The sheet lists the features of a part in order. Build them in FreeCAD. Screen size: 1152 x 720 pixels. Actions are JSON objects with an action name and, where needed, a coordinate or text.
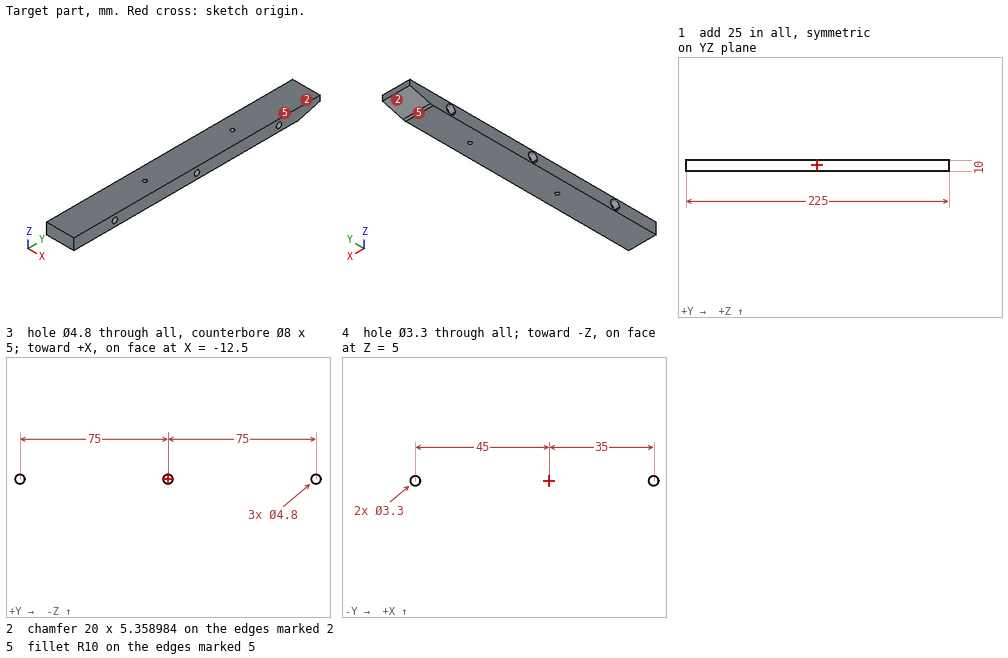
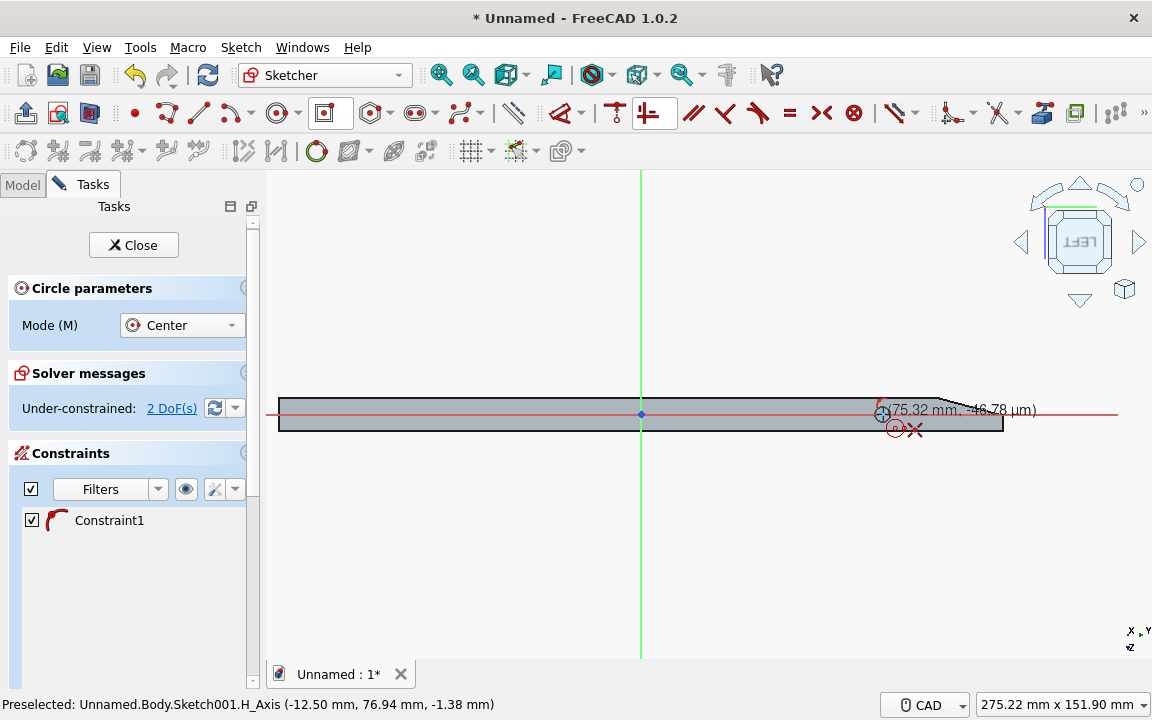
{"action": "scroll", "coordinate": [641, 414], "scroll_direction": "up", "scroll_amount": 6}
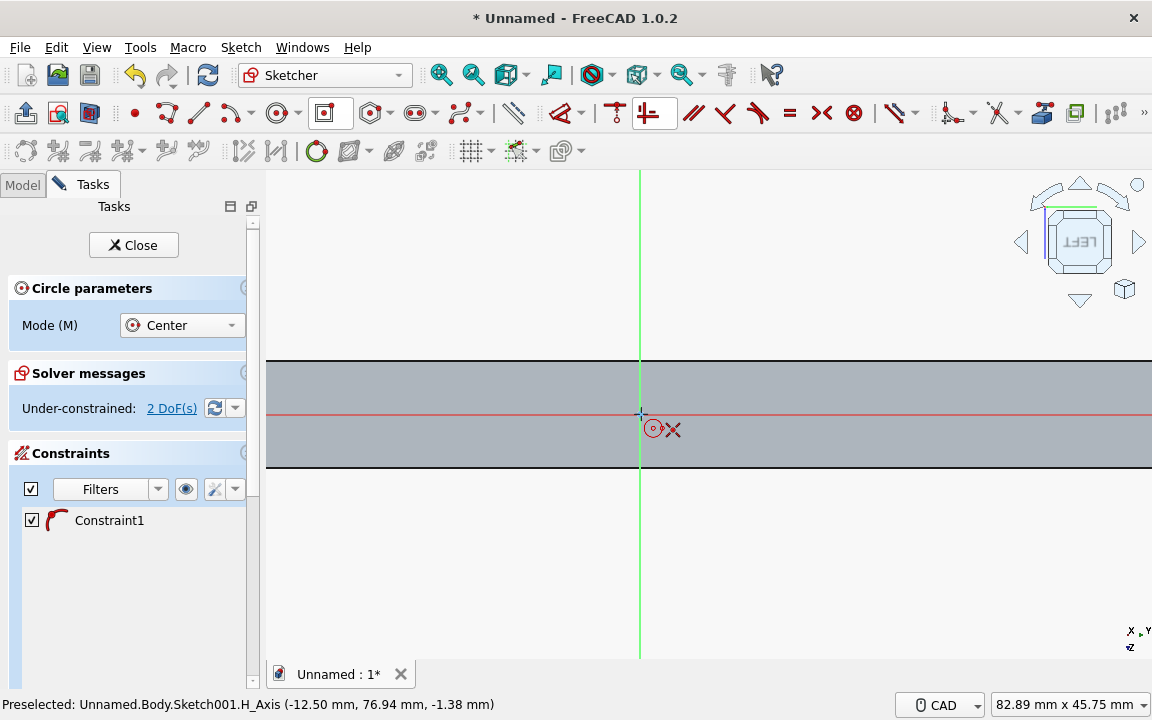
{"action": "left_click", "coordinate": [640, 414]}
{"action": "left_click", "coordinate": [658, 396]}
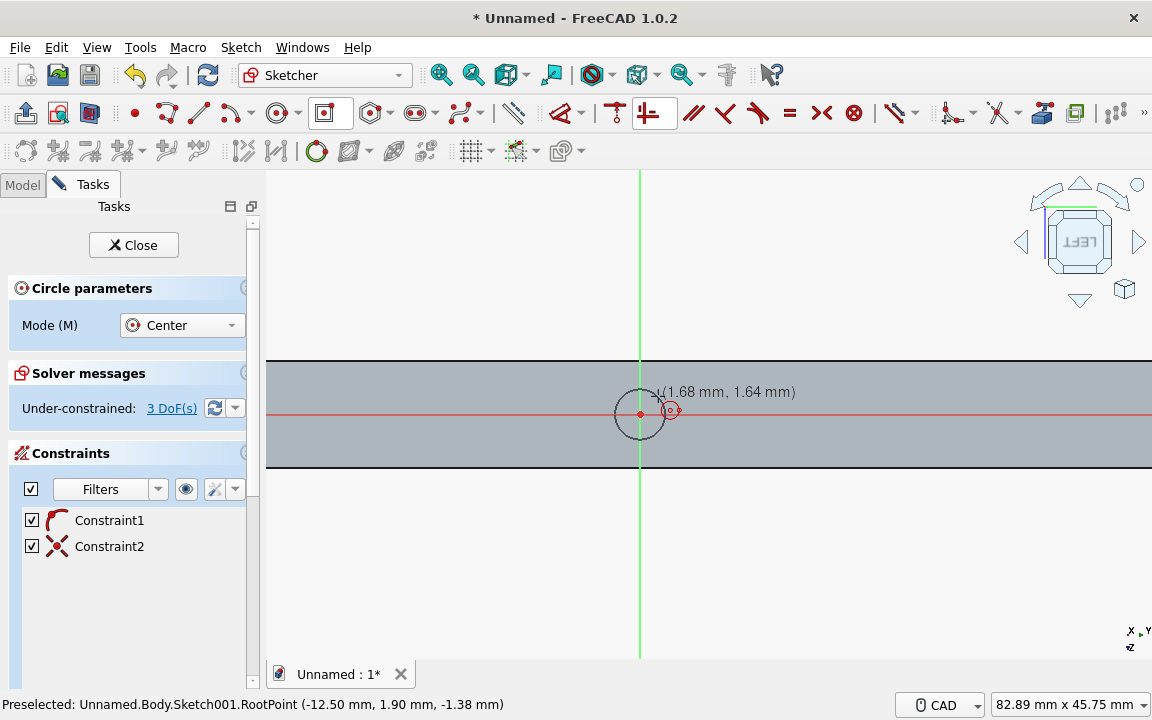
{"action": "scroll", "coordinate": [641, 414], "scroll_direction": "down", "scroll_amount": 6}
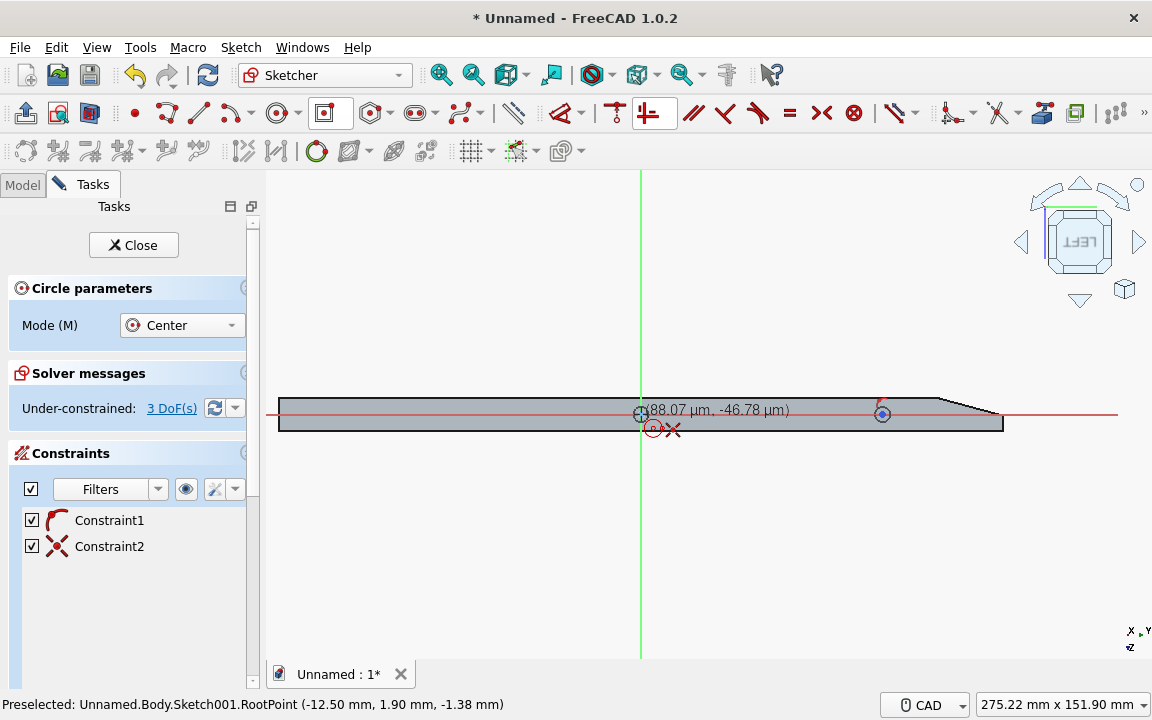
{"action": "scroll", "coordinate": [400, 414], "scroll_direction": "up", "scroll_amount": 6}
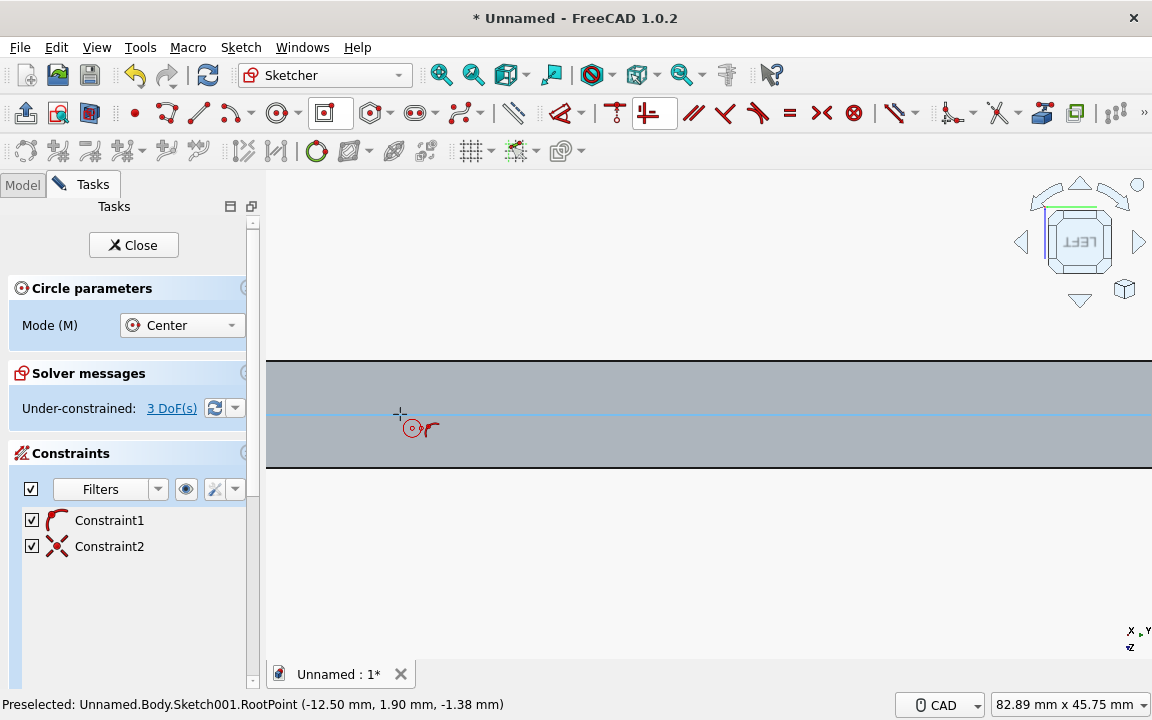
{"action": "left_click", "coordinate": [398, 414]}
{"action": "left_click", "coordinate": [416, 396]}
{"action": "key", "text": "Escape"}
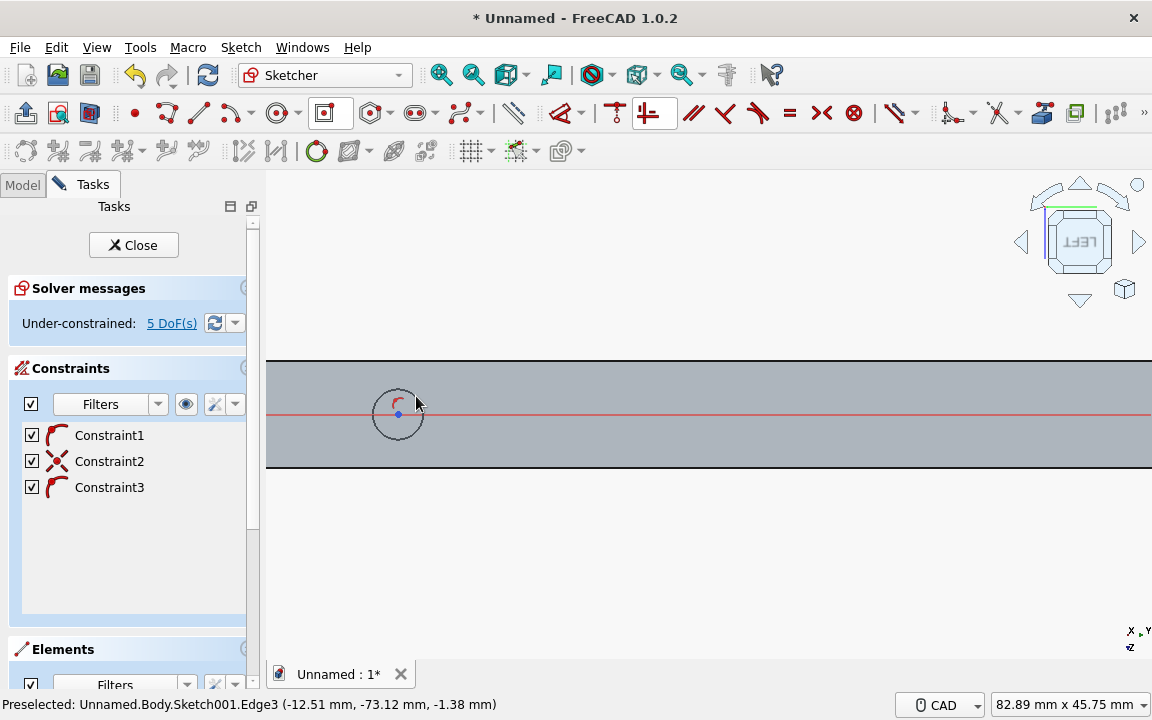
{"action": "scroll", "coordinate": [399, 414], "scroll_direction": "down", "scroll_amount": 6}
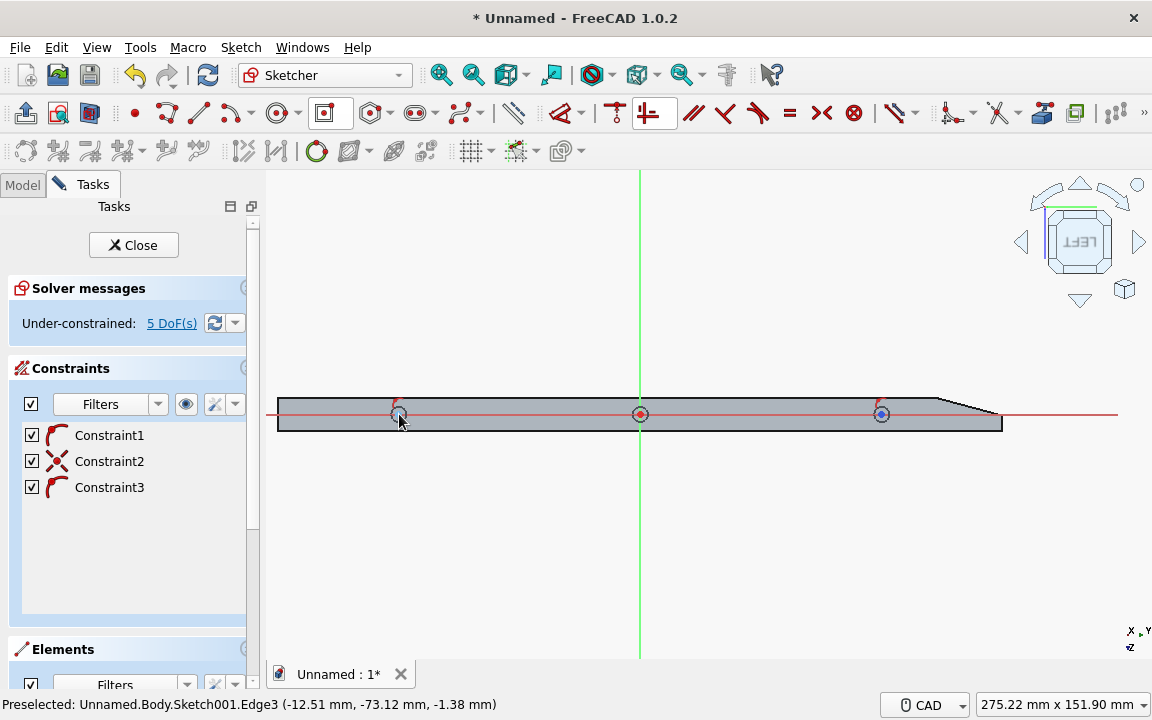
{"action": "scroll", "coordinate": [887, 409], "scroll_direction": "up", "scroll_amount": 5}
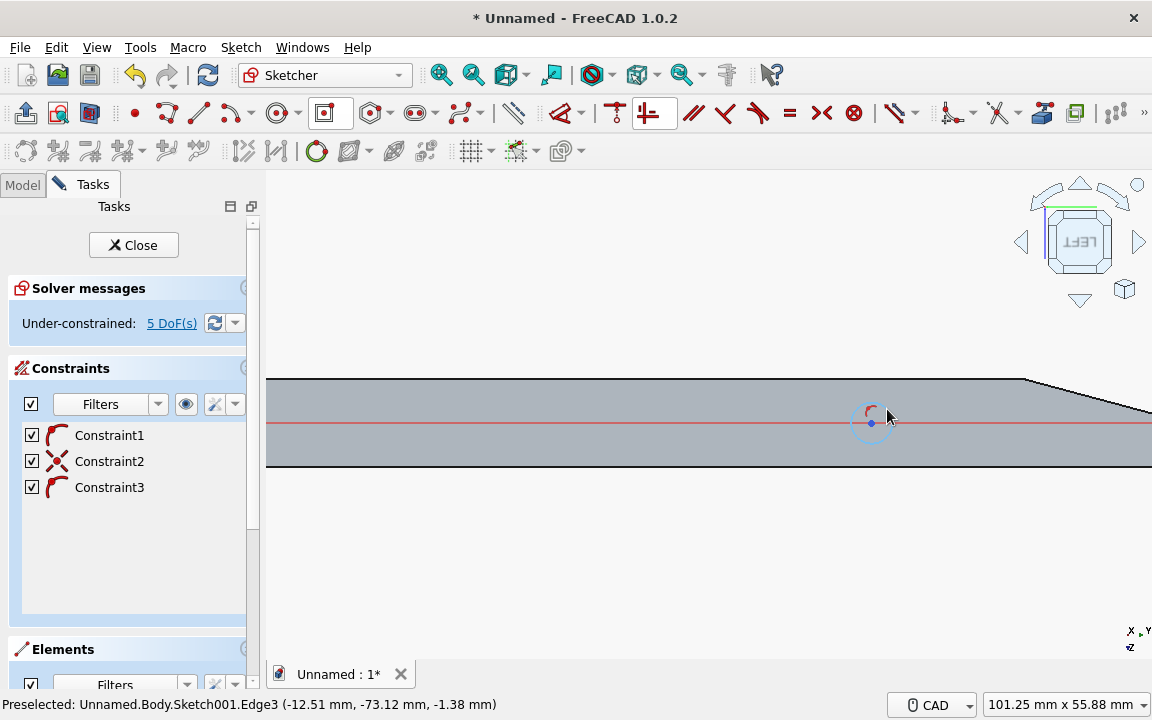
{"action": "left_click", "coordinate": [886, 409]}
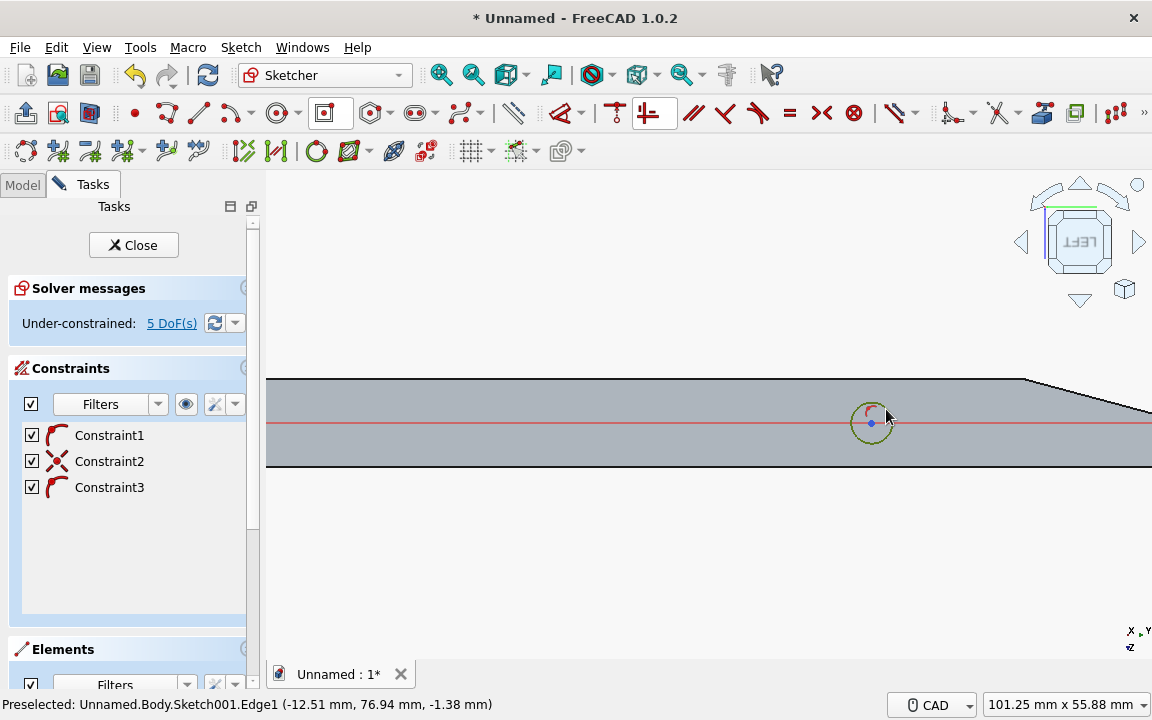
{"action": "scroll", "coordinate": [888, 409], "scroll_direction": "down", "scroll_amount": 5}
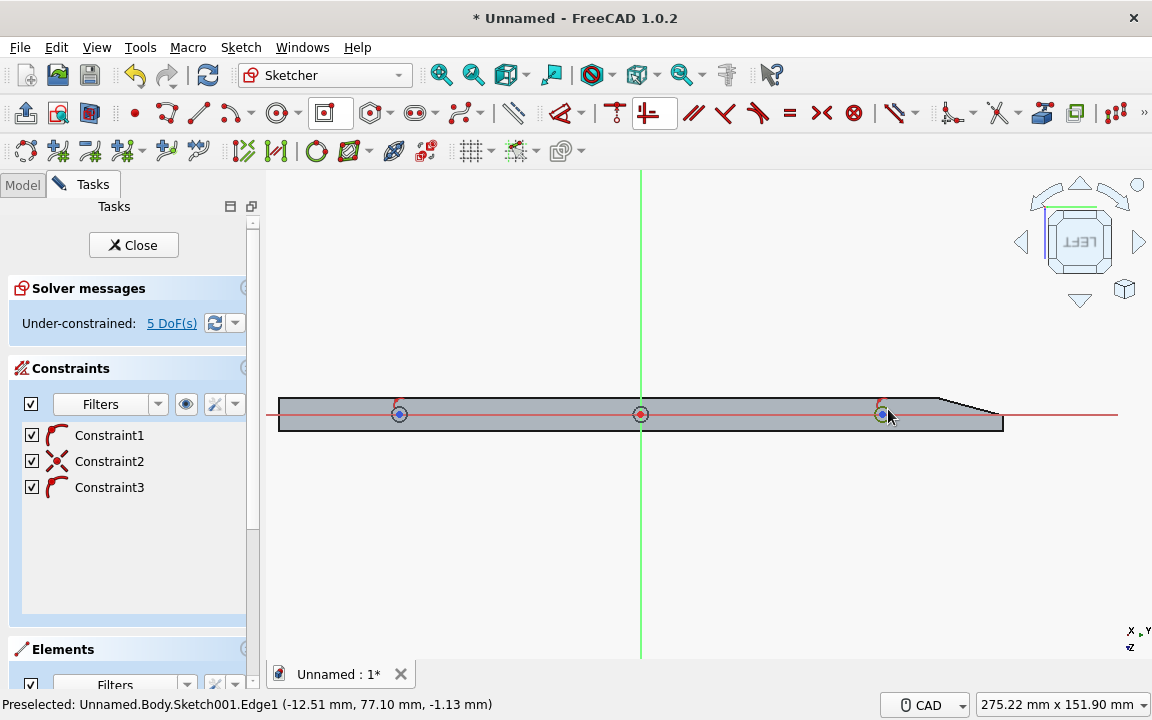
{"action": "scroll", "coordinate": [646, 409], "scroll_direction": "up", "scroll_amount": 5}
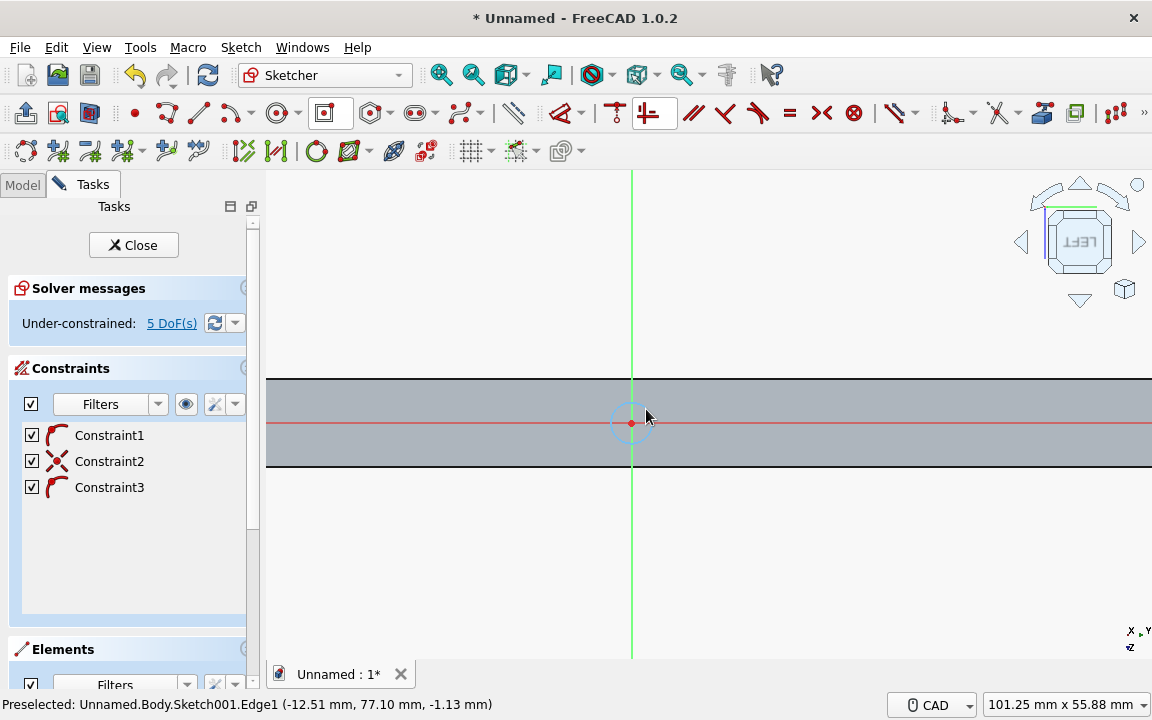
{"action": "left_click", "coordinate": [646, 409]}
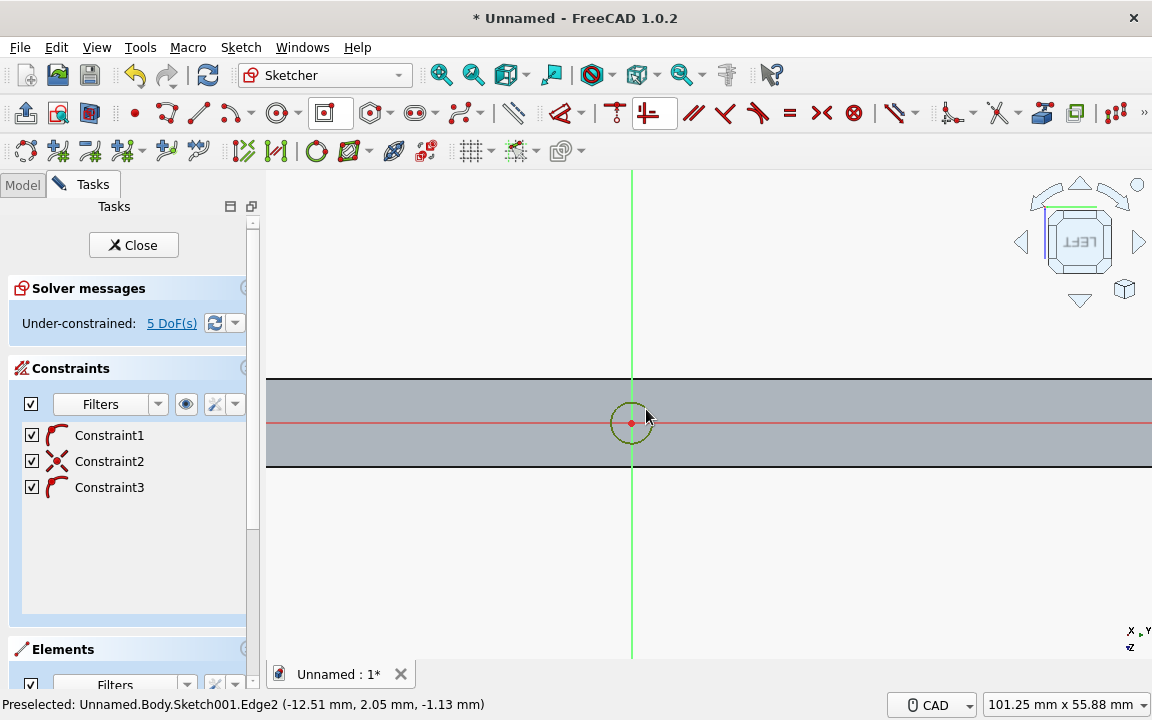
{"action": "scroll", "coordinate": [646, 409], "scroll_direction": "down", "scroll_amount": 5}